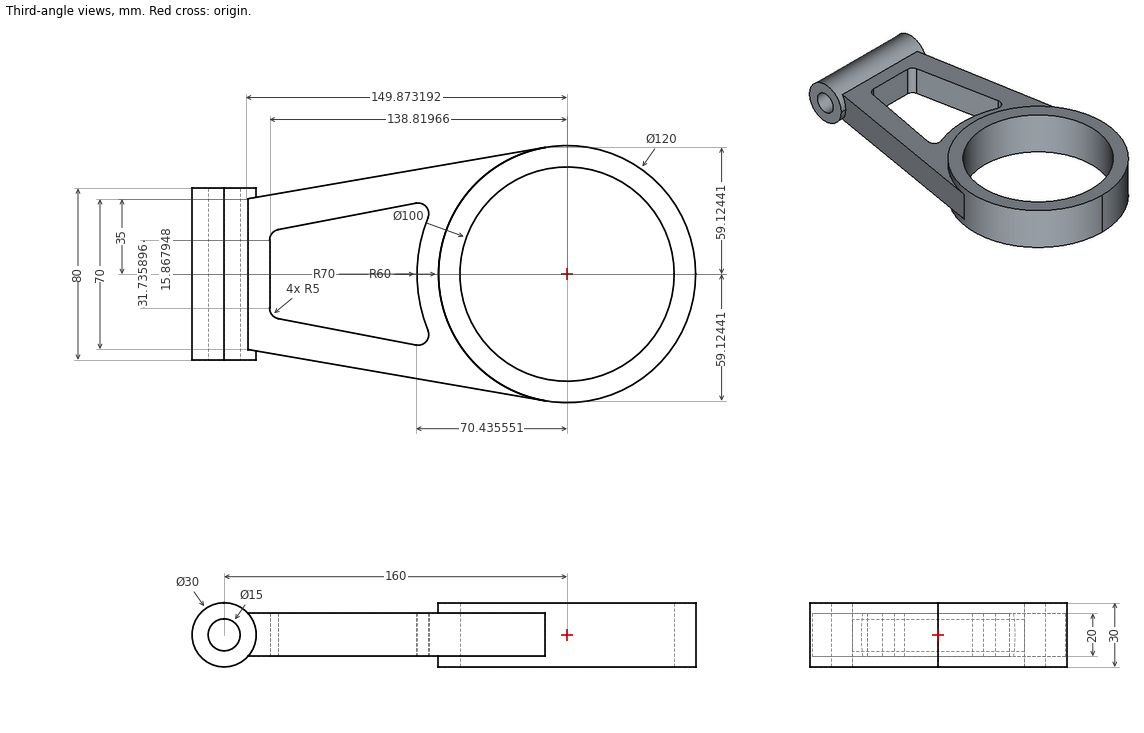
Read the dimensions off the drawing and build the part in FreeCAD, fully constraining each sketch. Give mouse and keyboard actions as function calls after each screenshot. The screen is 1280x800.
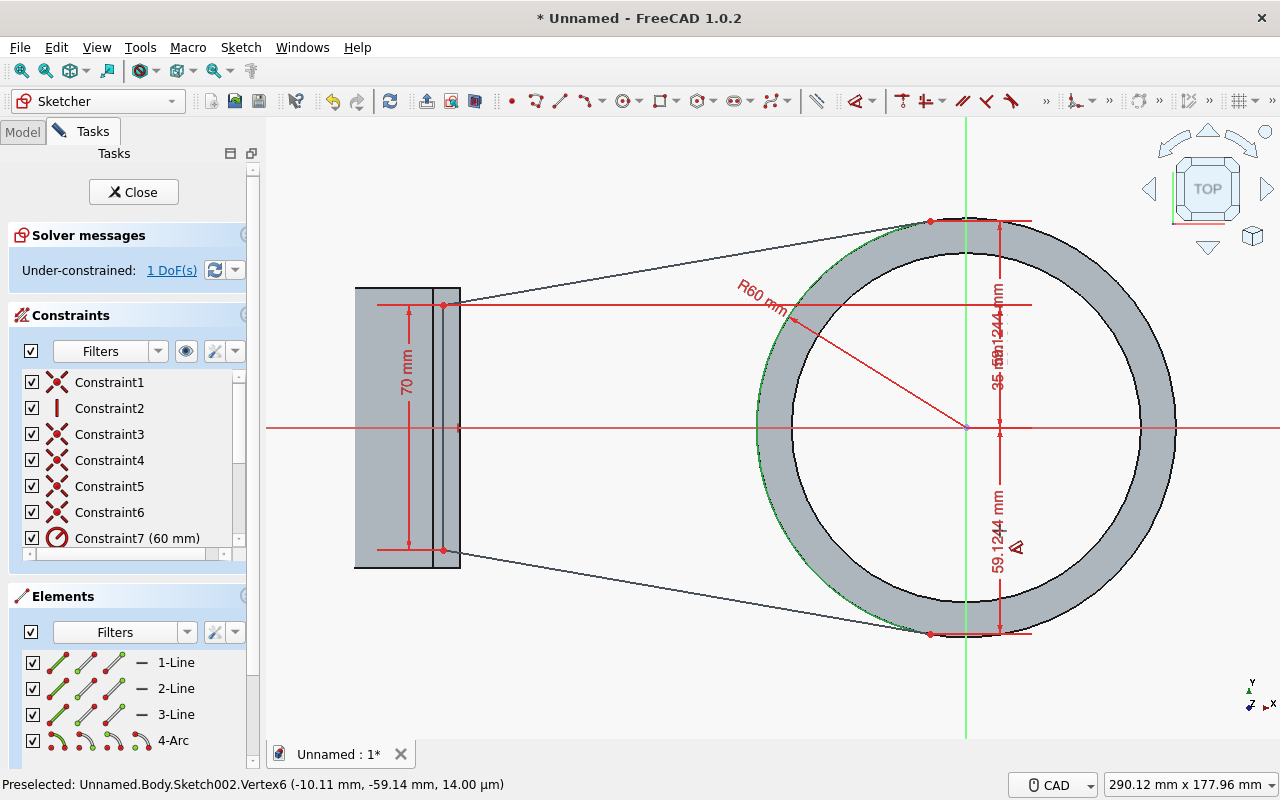
click(443, 305)
click(522, 271)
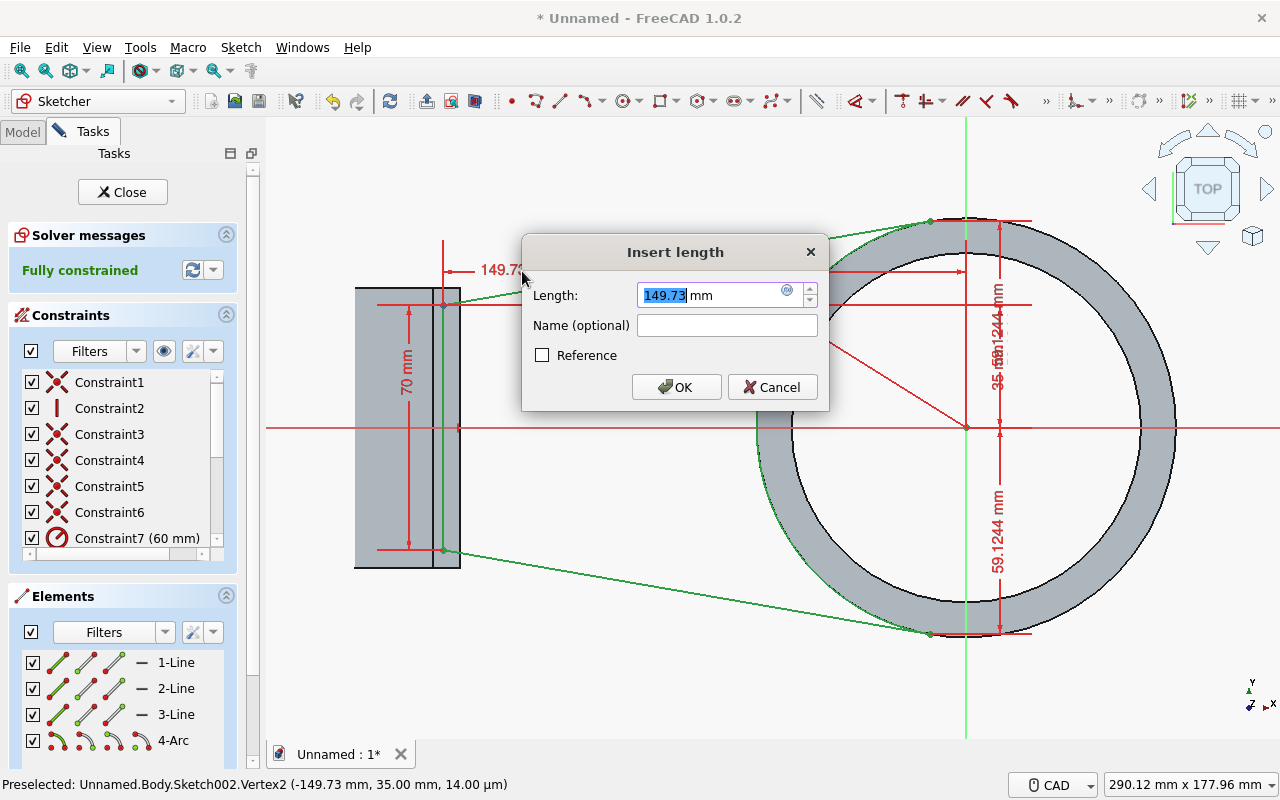
text(149.873192)
key(Return)
key(Escape)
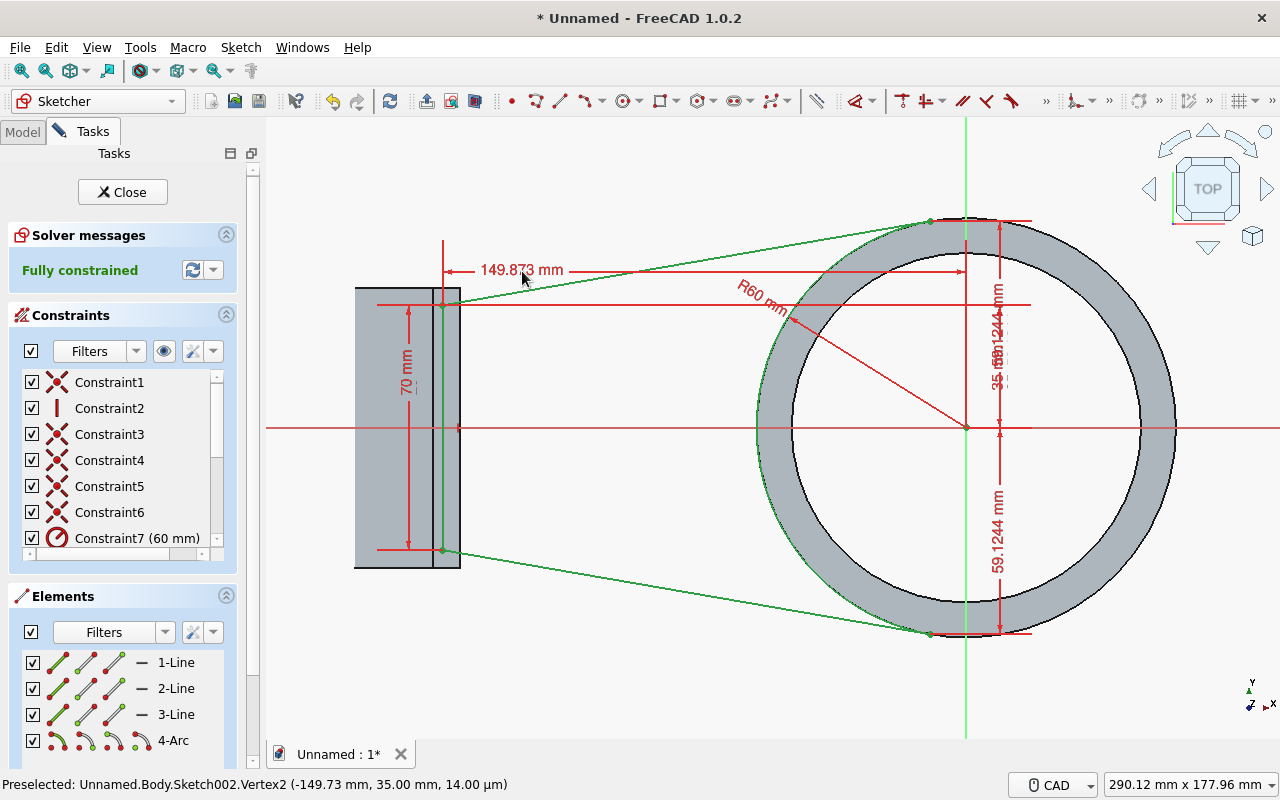
click(123, 192)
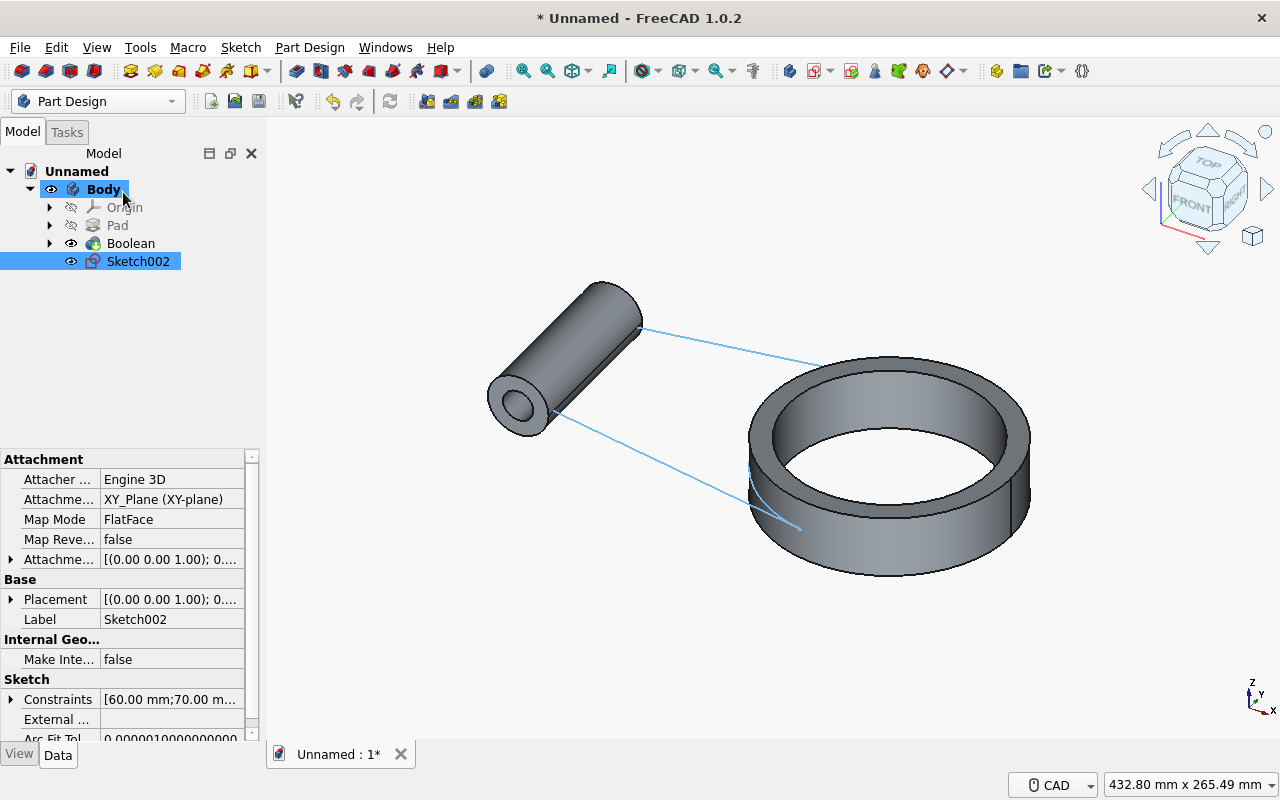
click(132, 72)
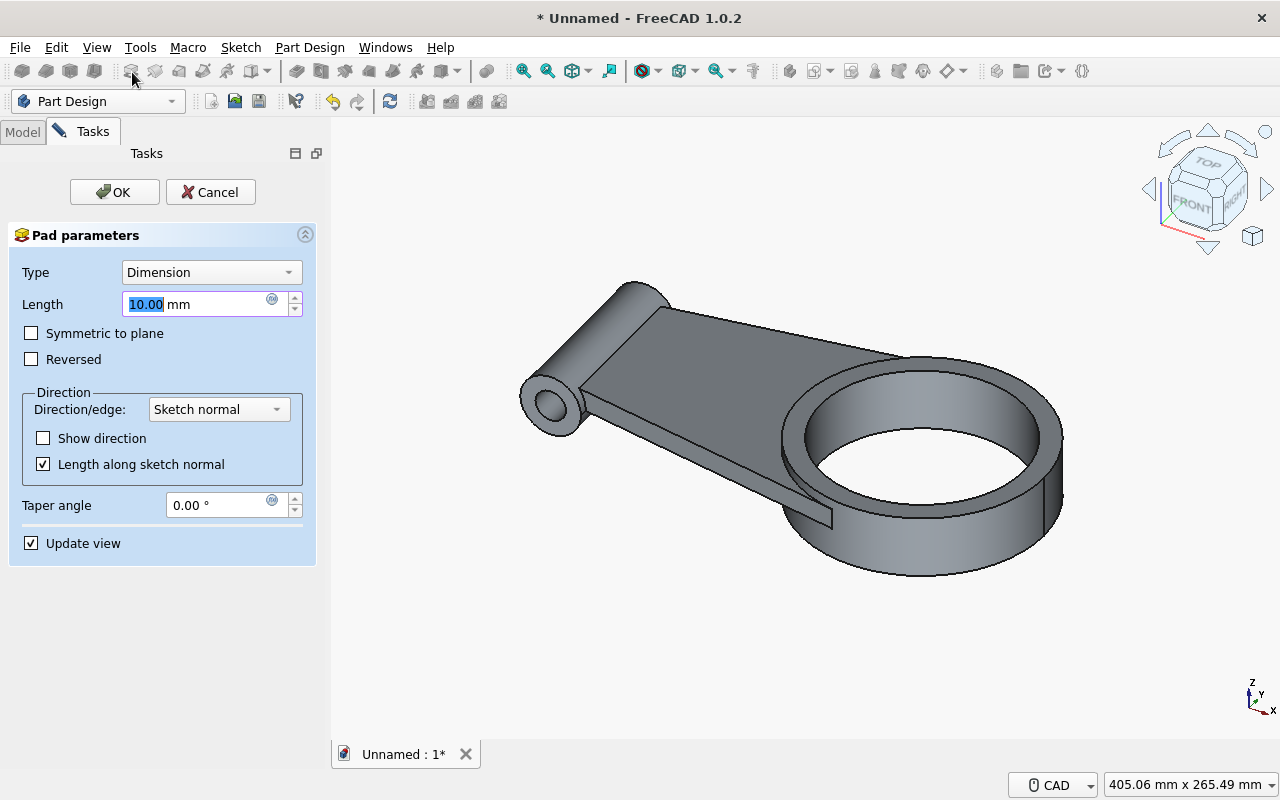
text(20)
key(Tab)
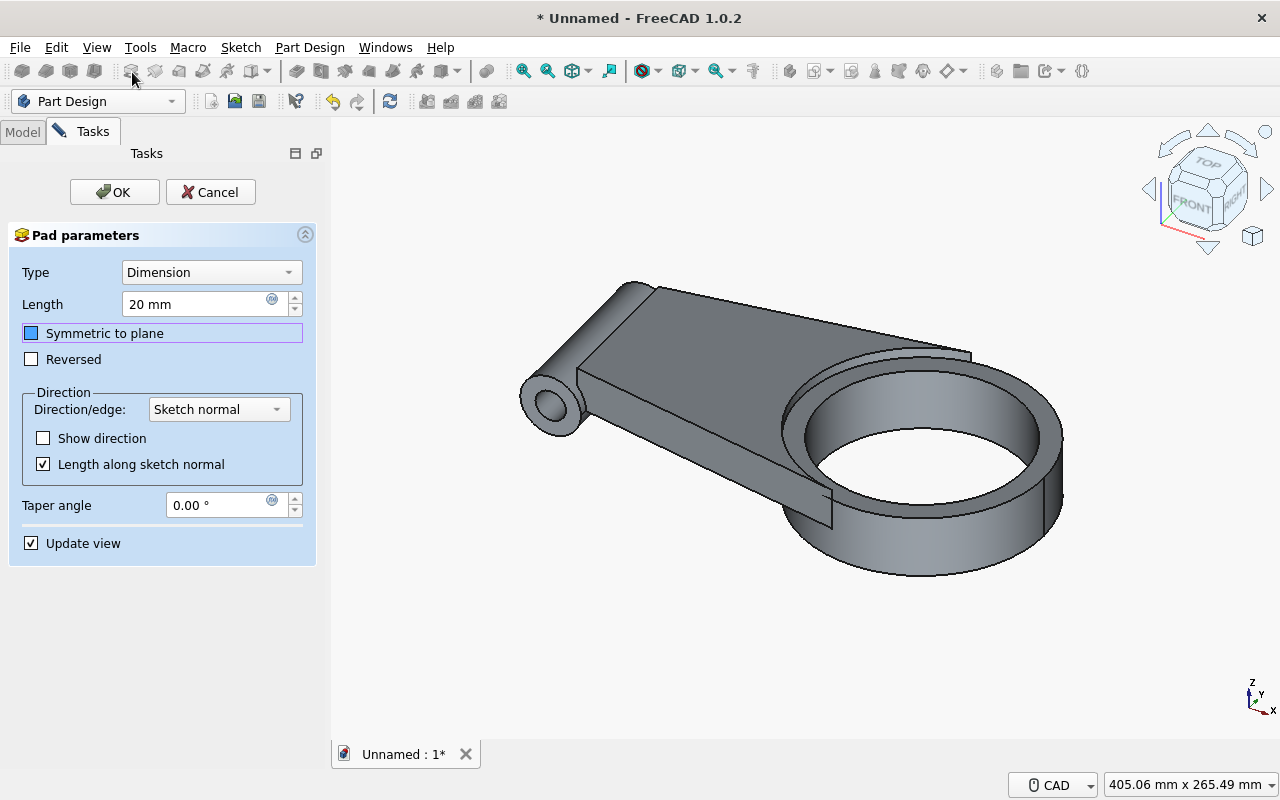
click(30, 333)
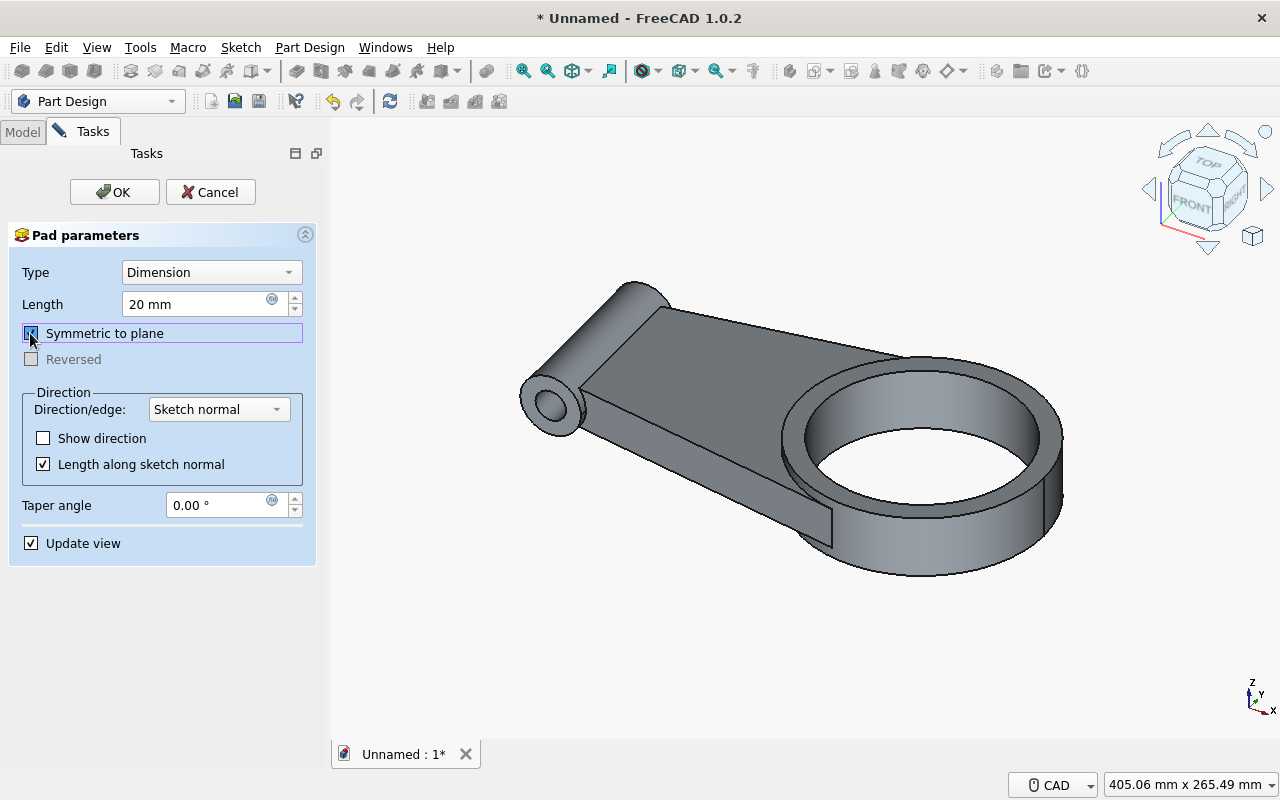
click(115, 192)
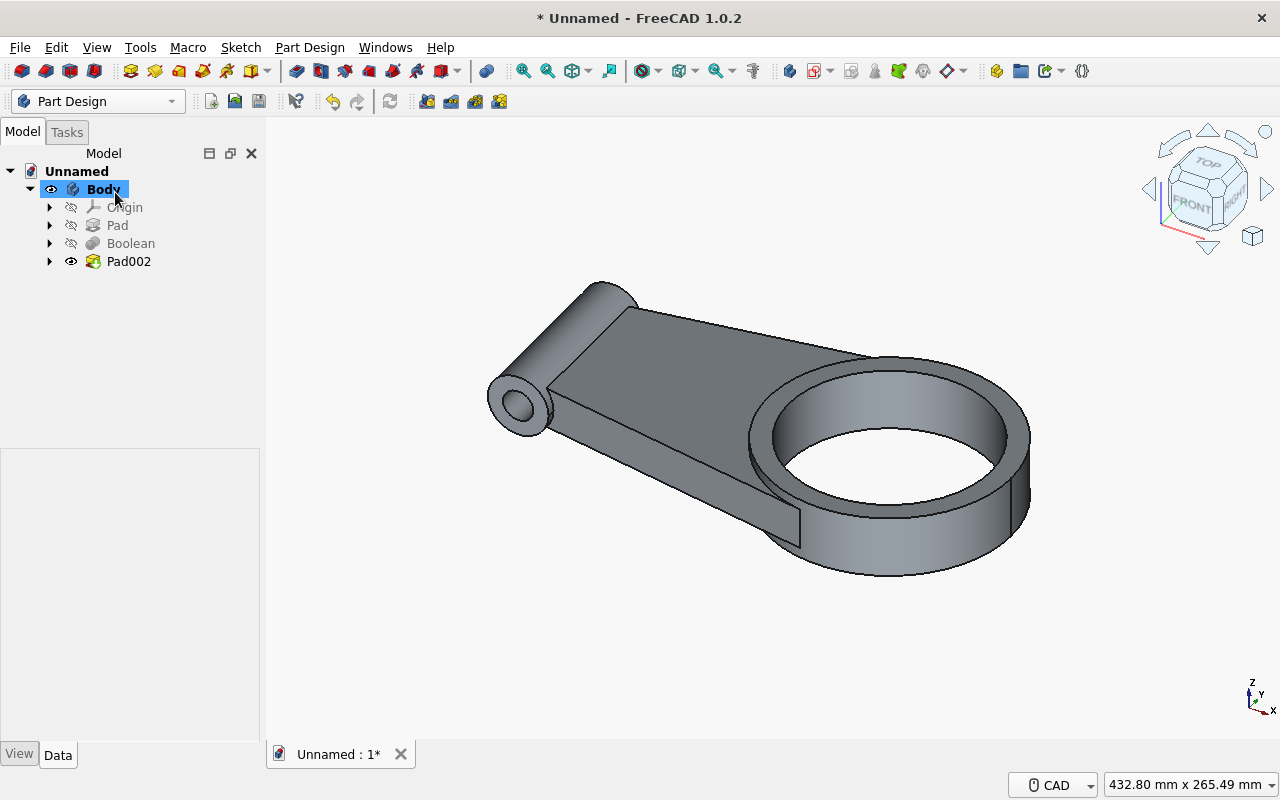
click(688, 380)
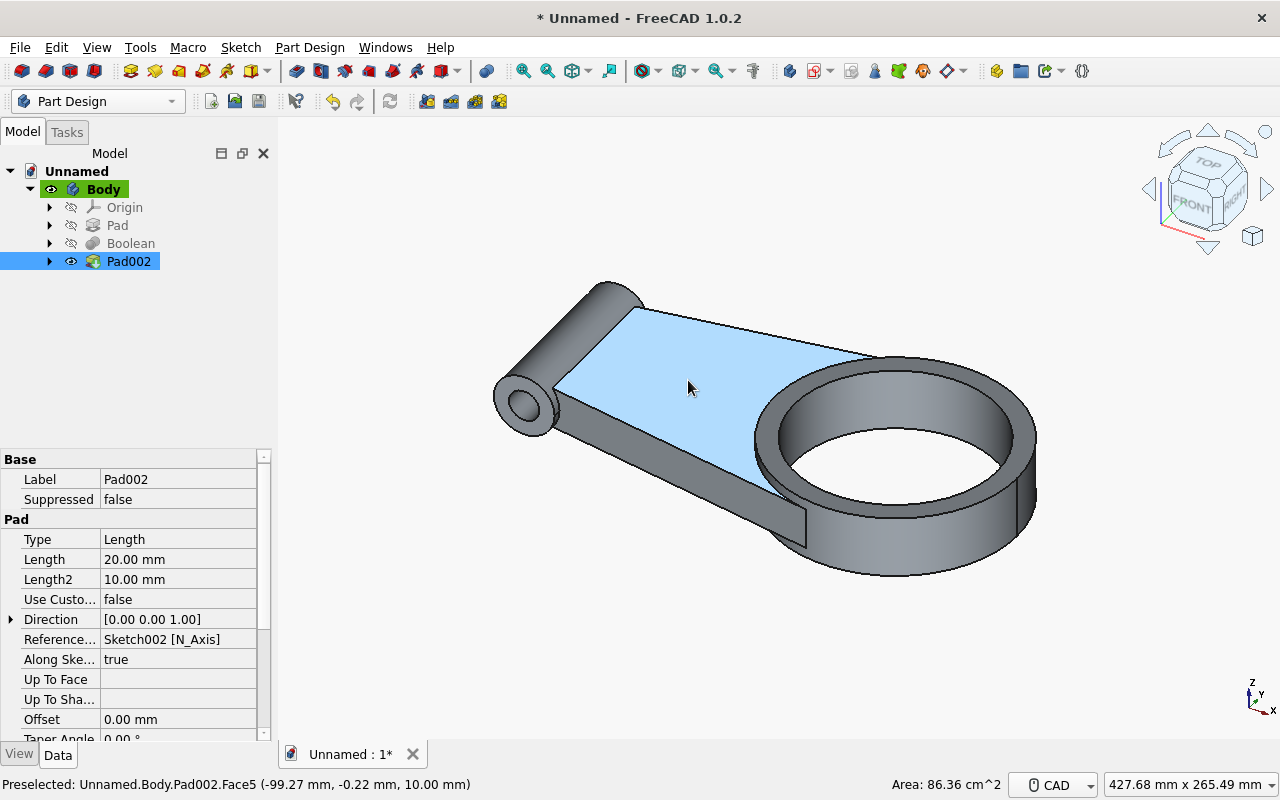
click(814, 72)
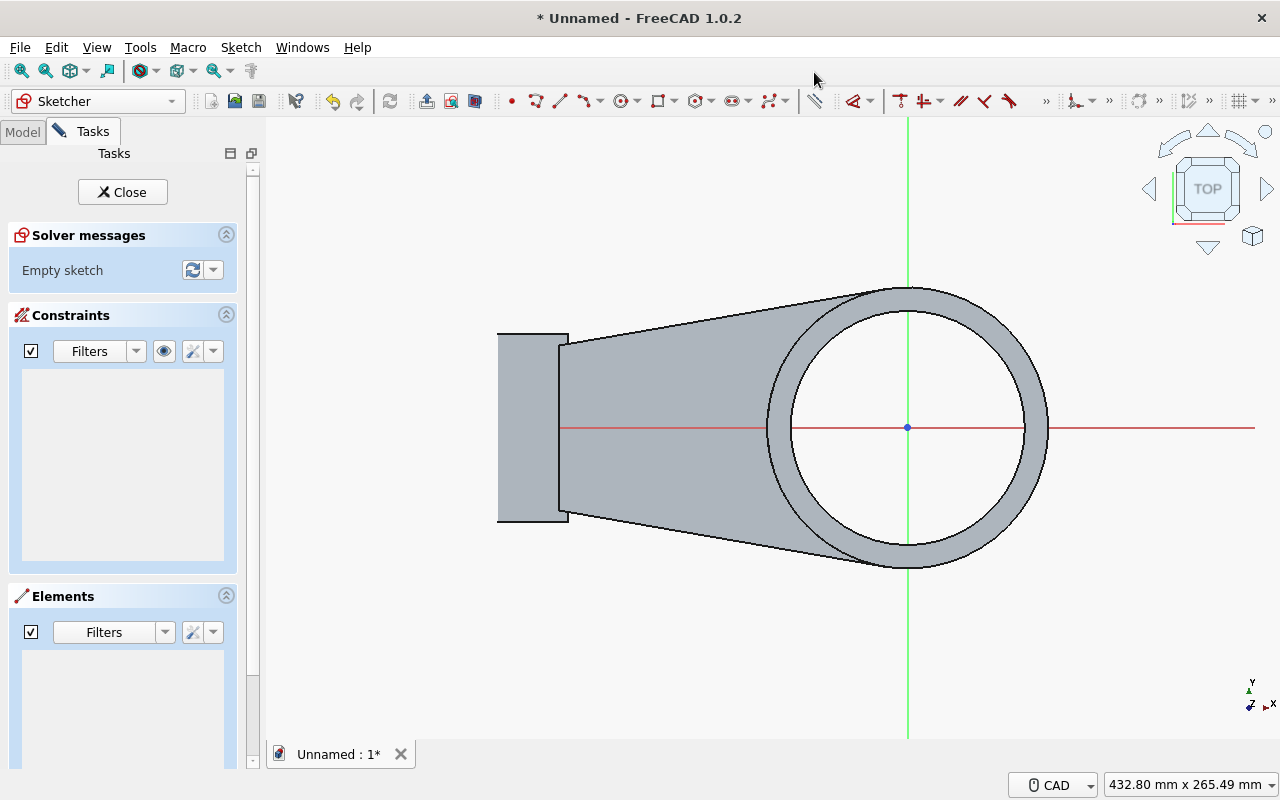
scroll(794, 428, up, 3)